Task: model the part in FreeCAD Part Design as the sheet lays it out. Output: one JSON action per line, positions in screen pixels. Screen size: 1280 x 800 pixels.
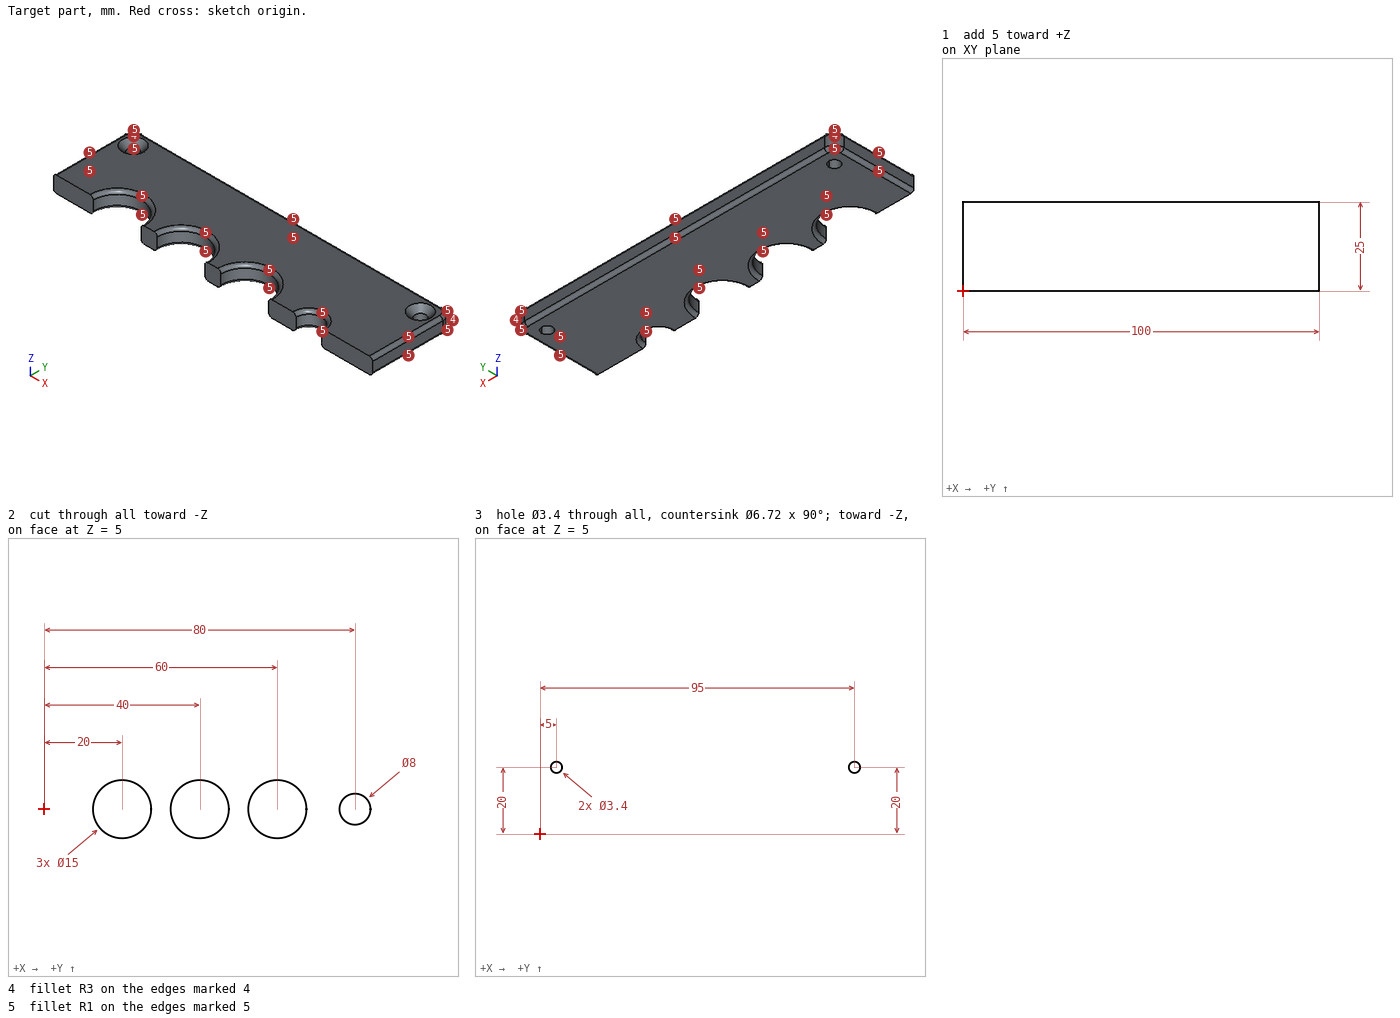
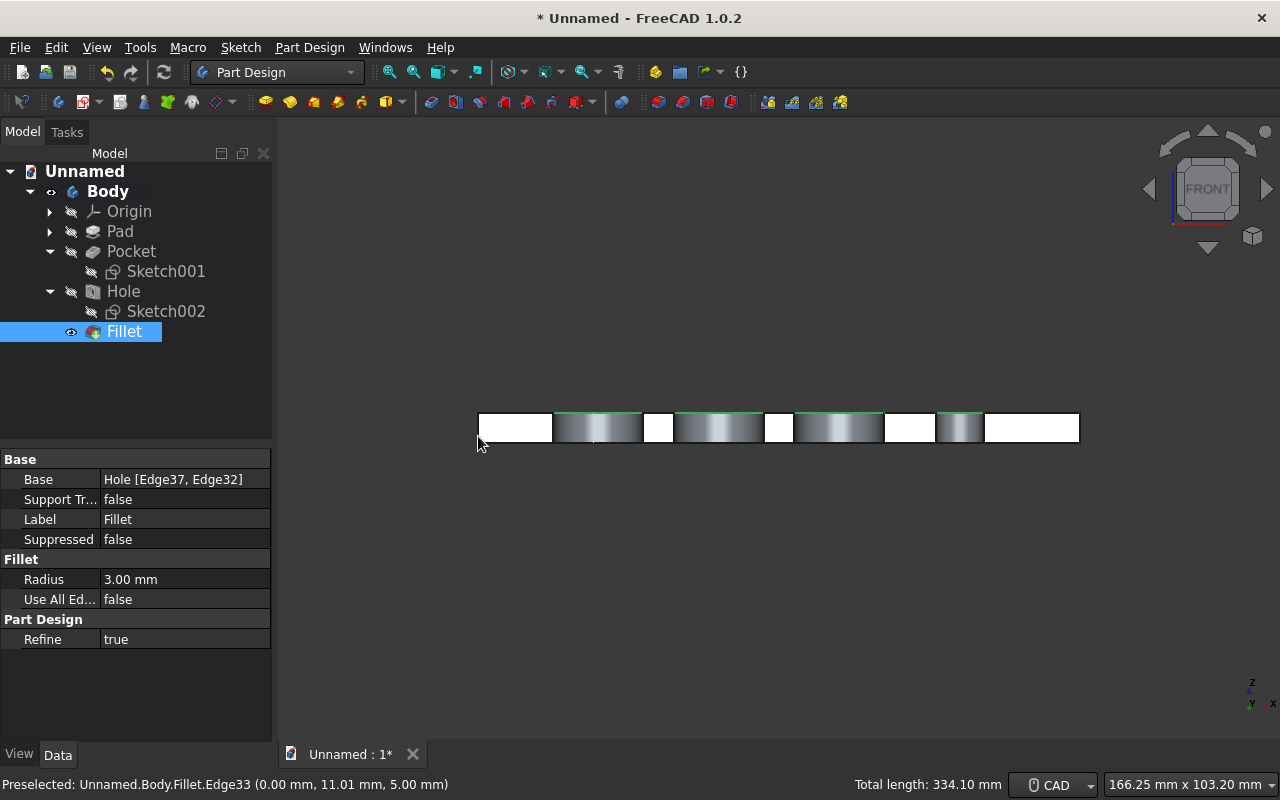
{"action": "left_click", "coordinate": [598, 442], "text": "ctrl"}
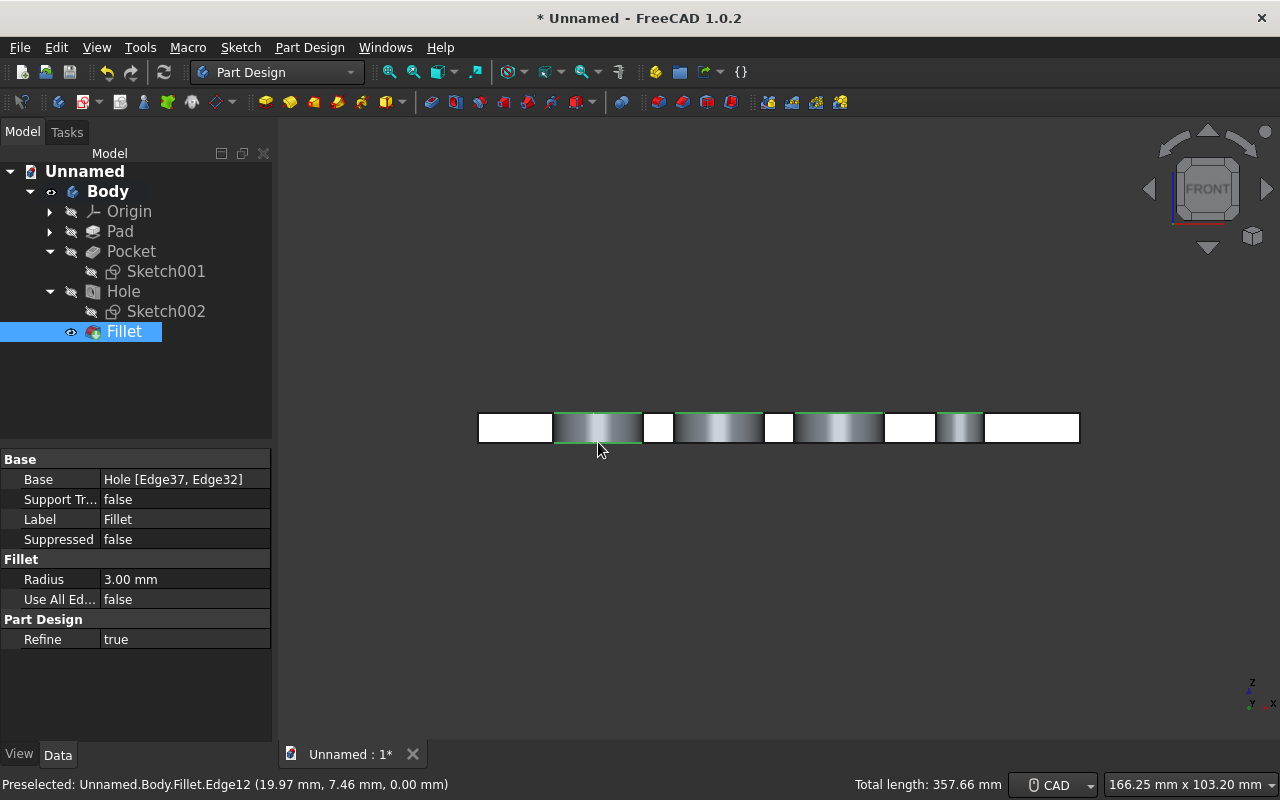
{"action": "left_click", "coordinate": [719, 442], "text": "ctrl"}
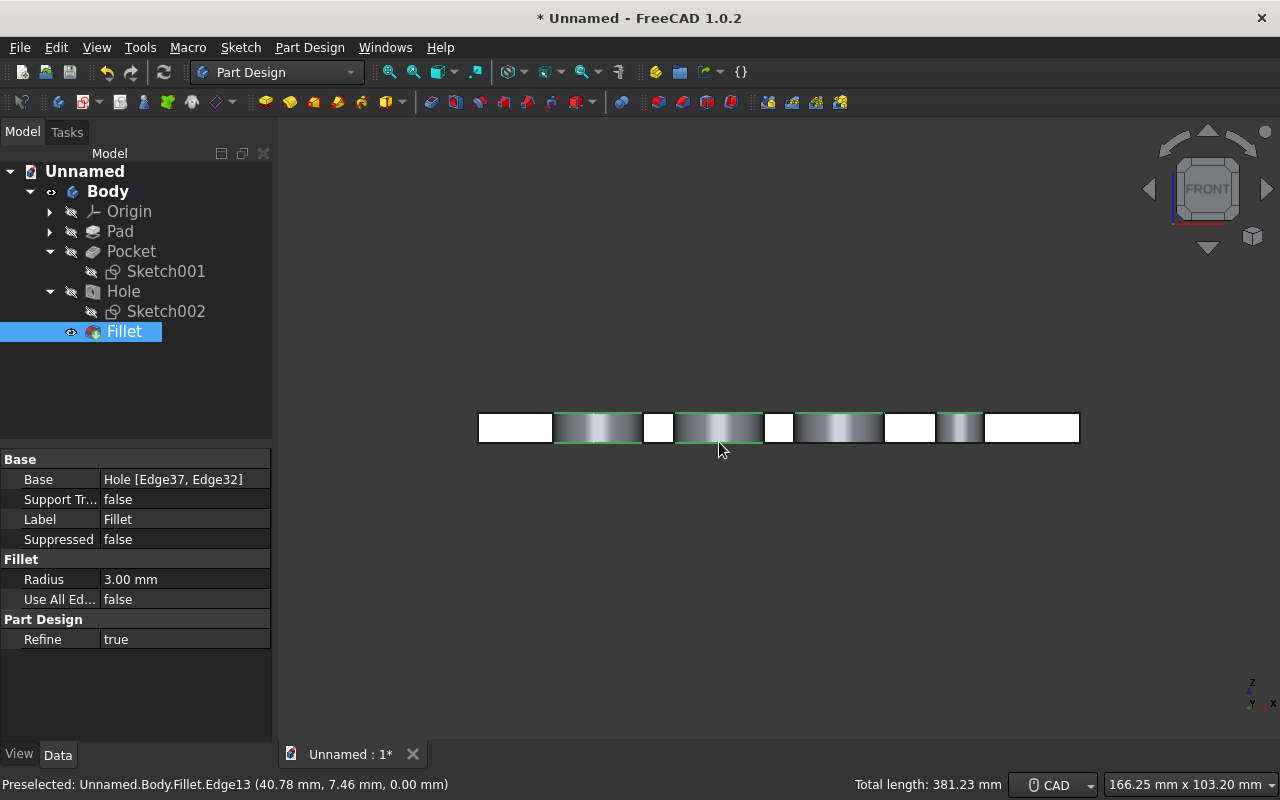
{"action": "left_click", "coordinate": [839, 442], "text": "ctrl"}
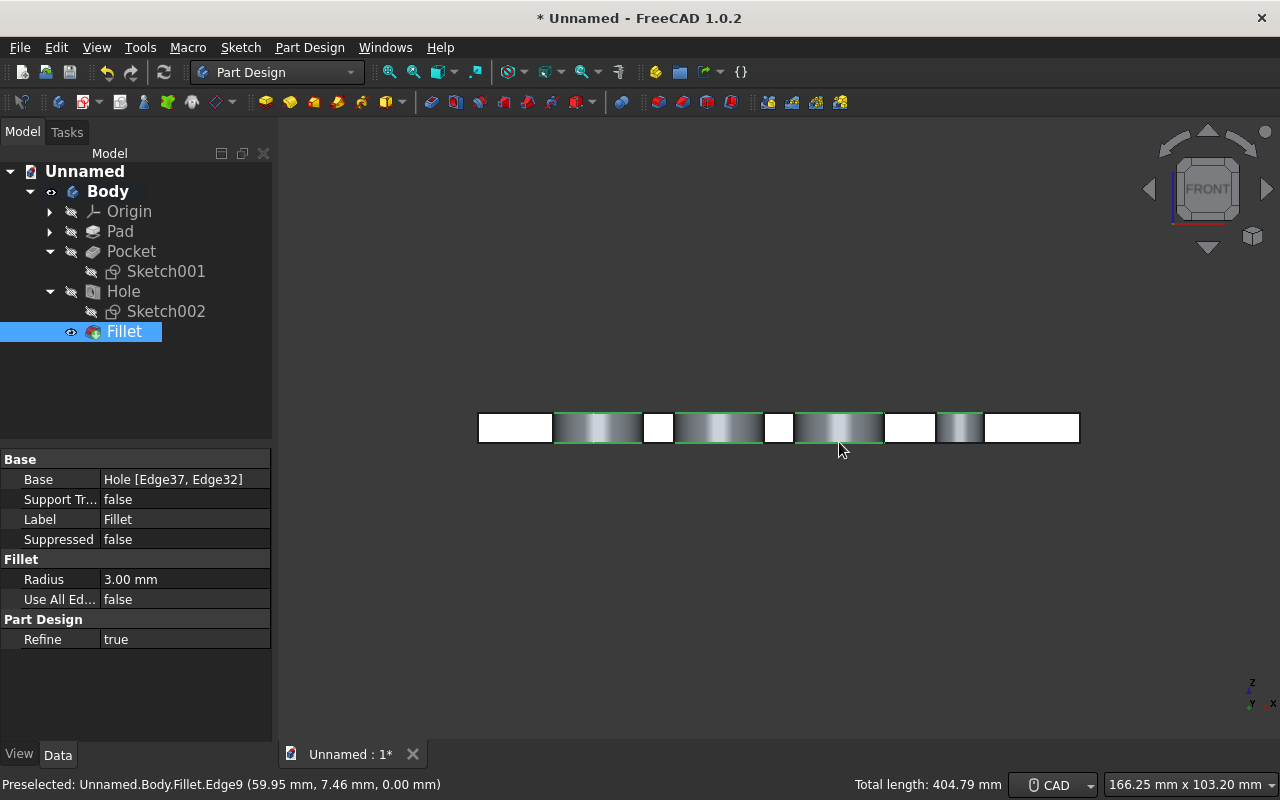
{"action": "left_click", "coordinate": [960, 442], "text": "ctrl"}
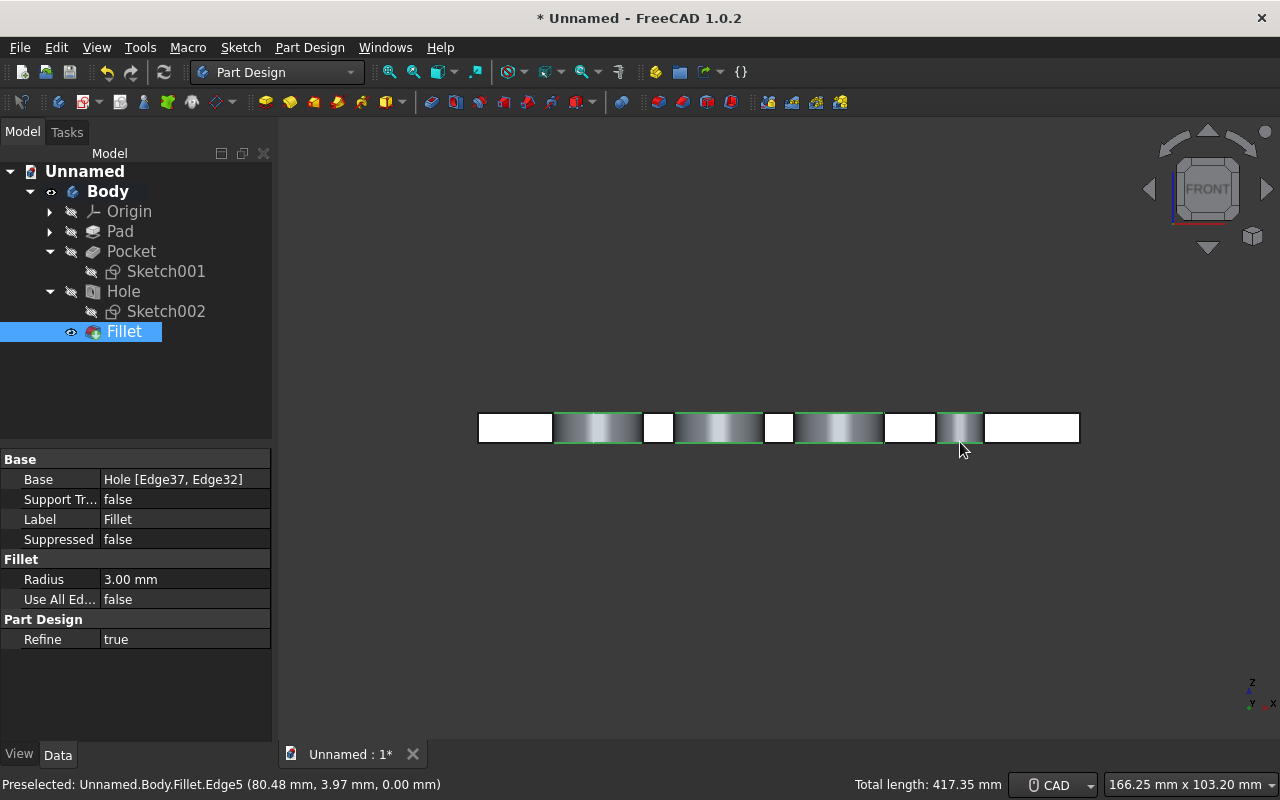
{"action": "key", "text": "3"}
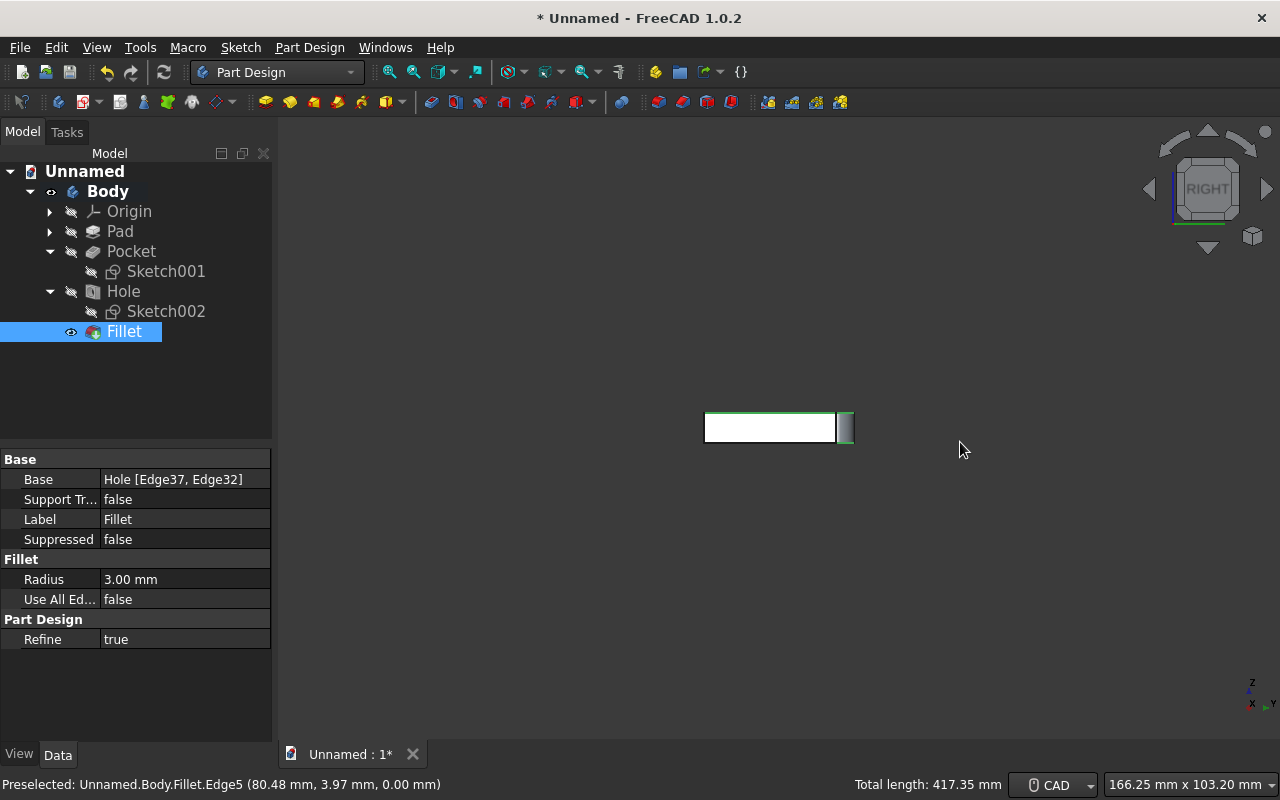
{"action": "left_click", "coordinate": [390, 72]}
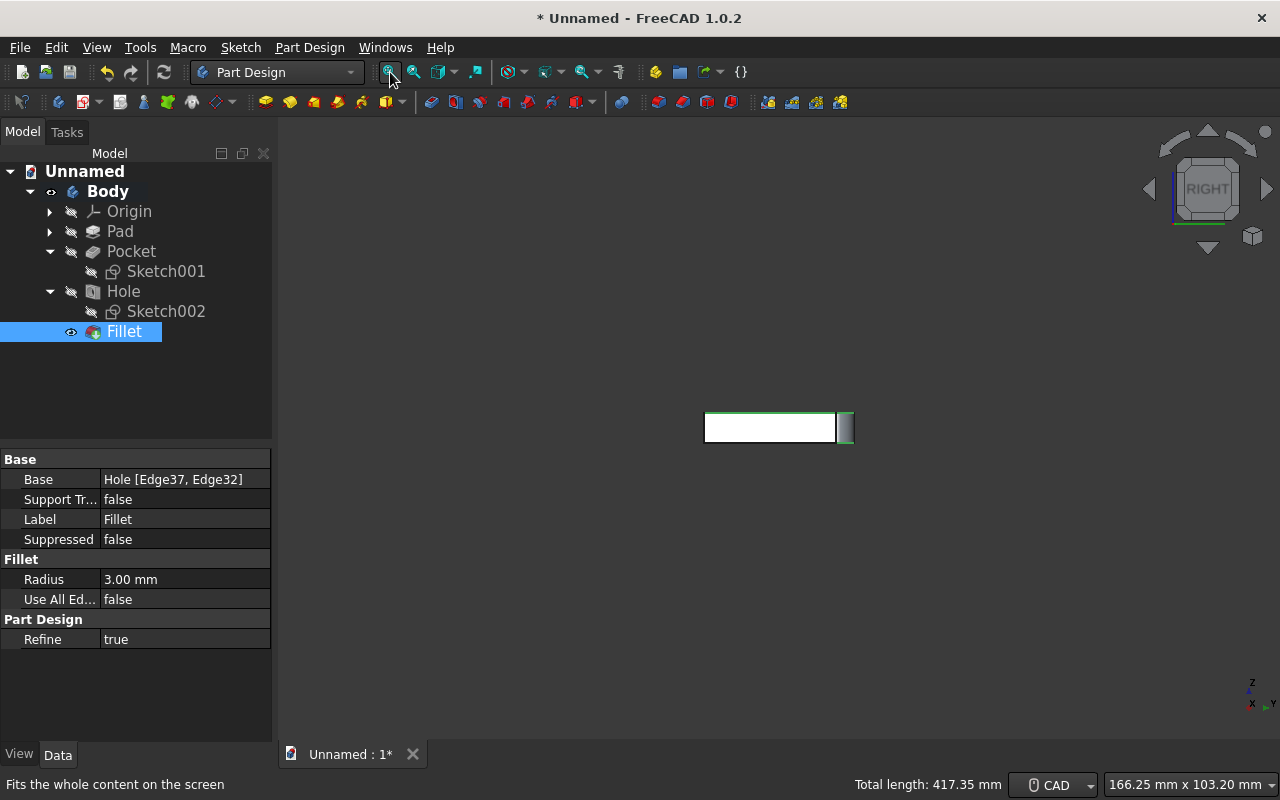
{"action": "left_click", "coordinate": [770, 442], "text": "ctrl"}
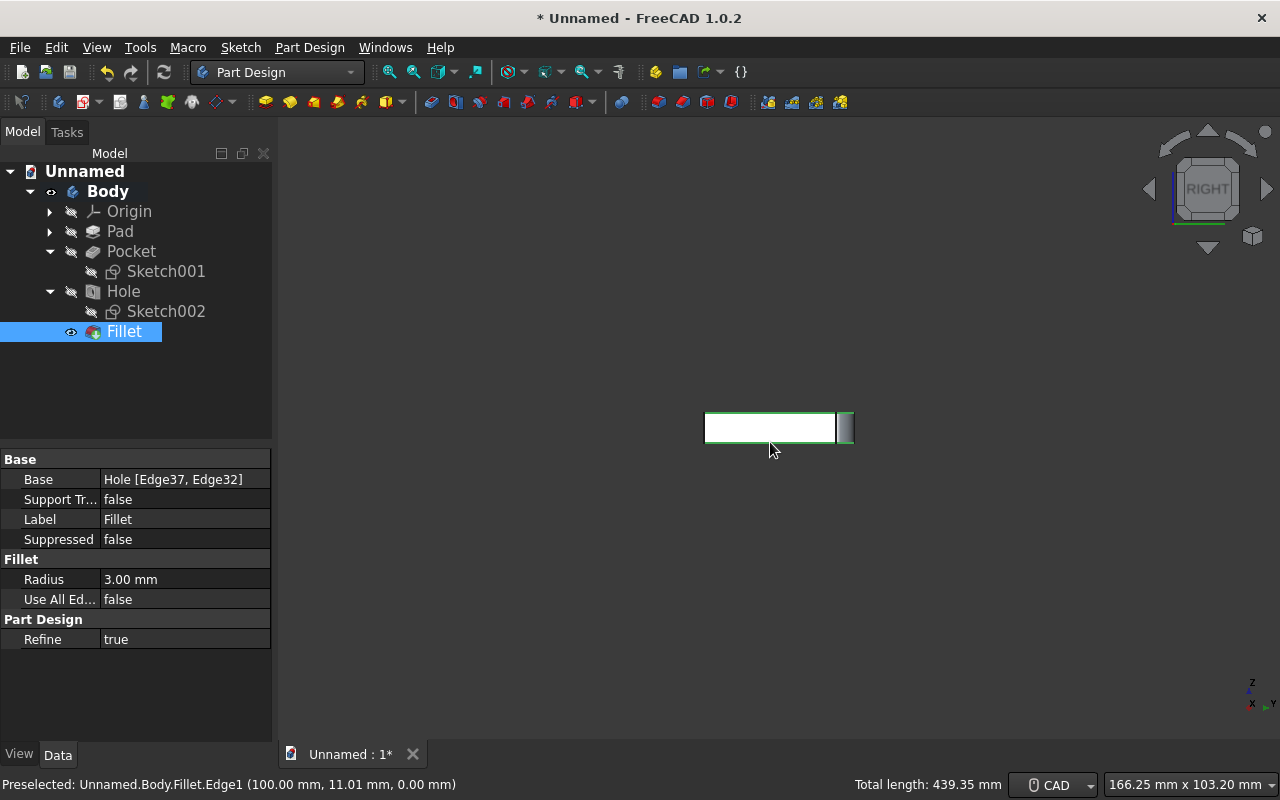
{"action": "key", "text": "5"}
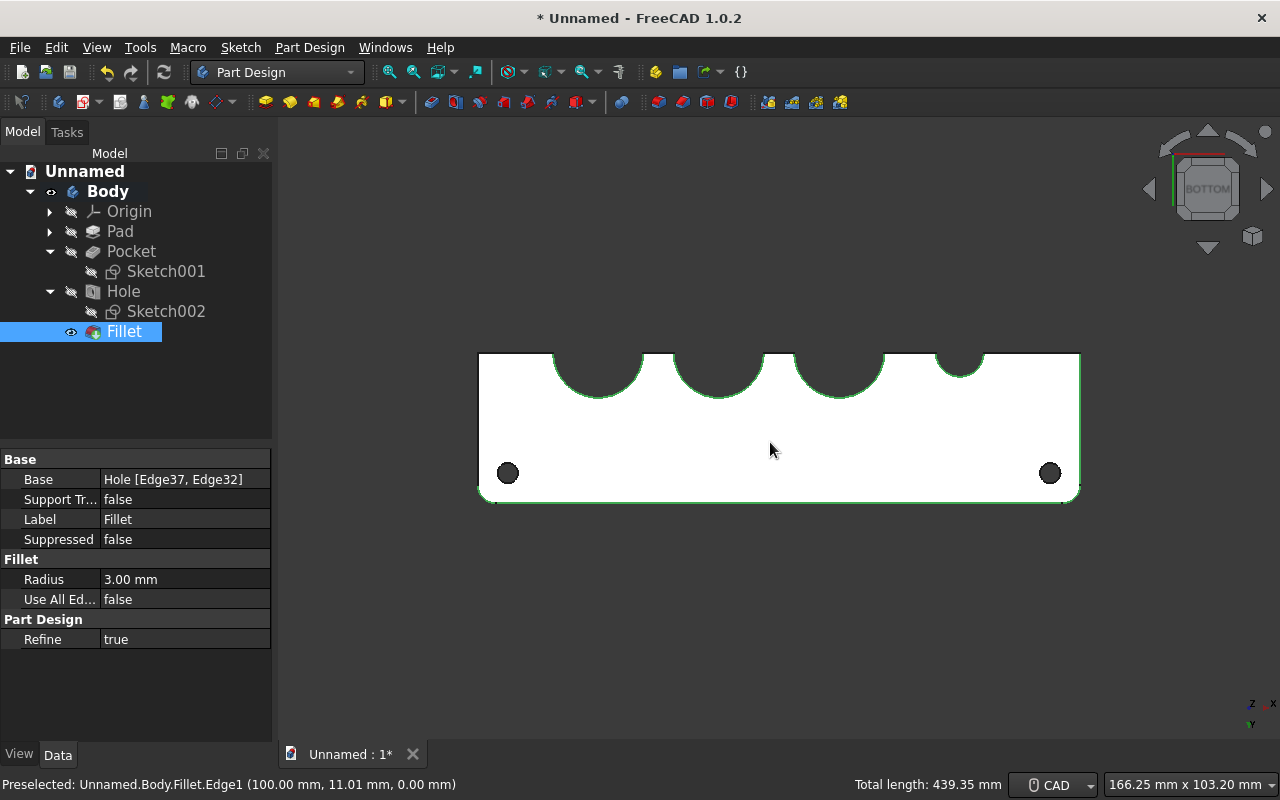
{"action": "left_click", "coordinate": [478, 418], "text": "ctrl"}